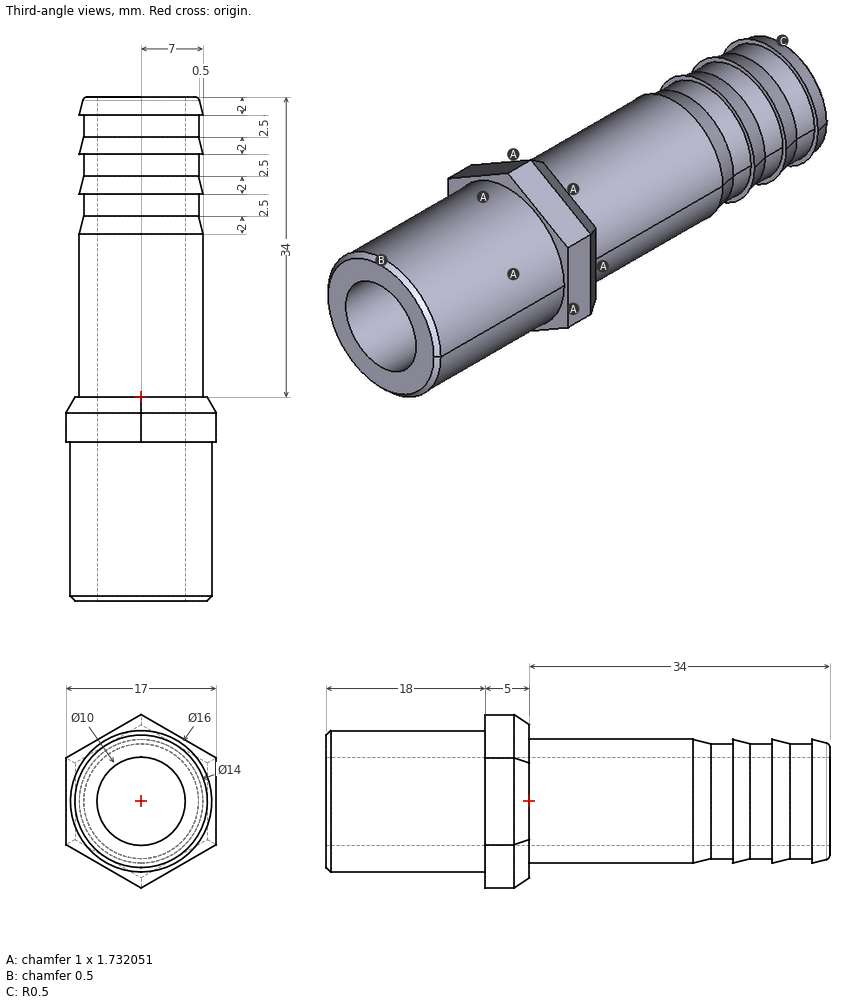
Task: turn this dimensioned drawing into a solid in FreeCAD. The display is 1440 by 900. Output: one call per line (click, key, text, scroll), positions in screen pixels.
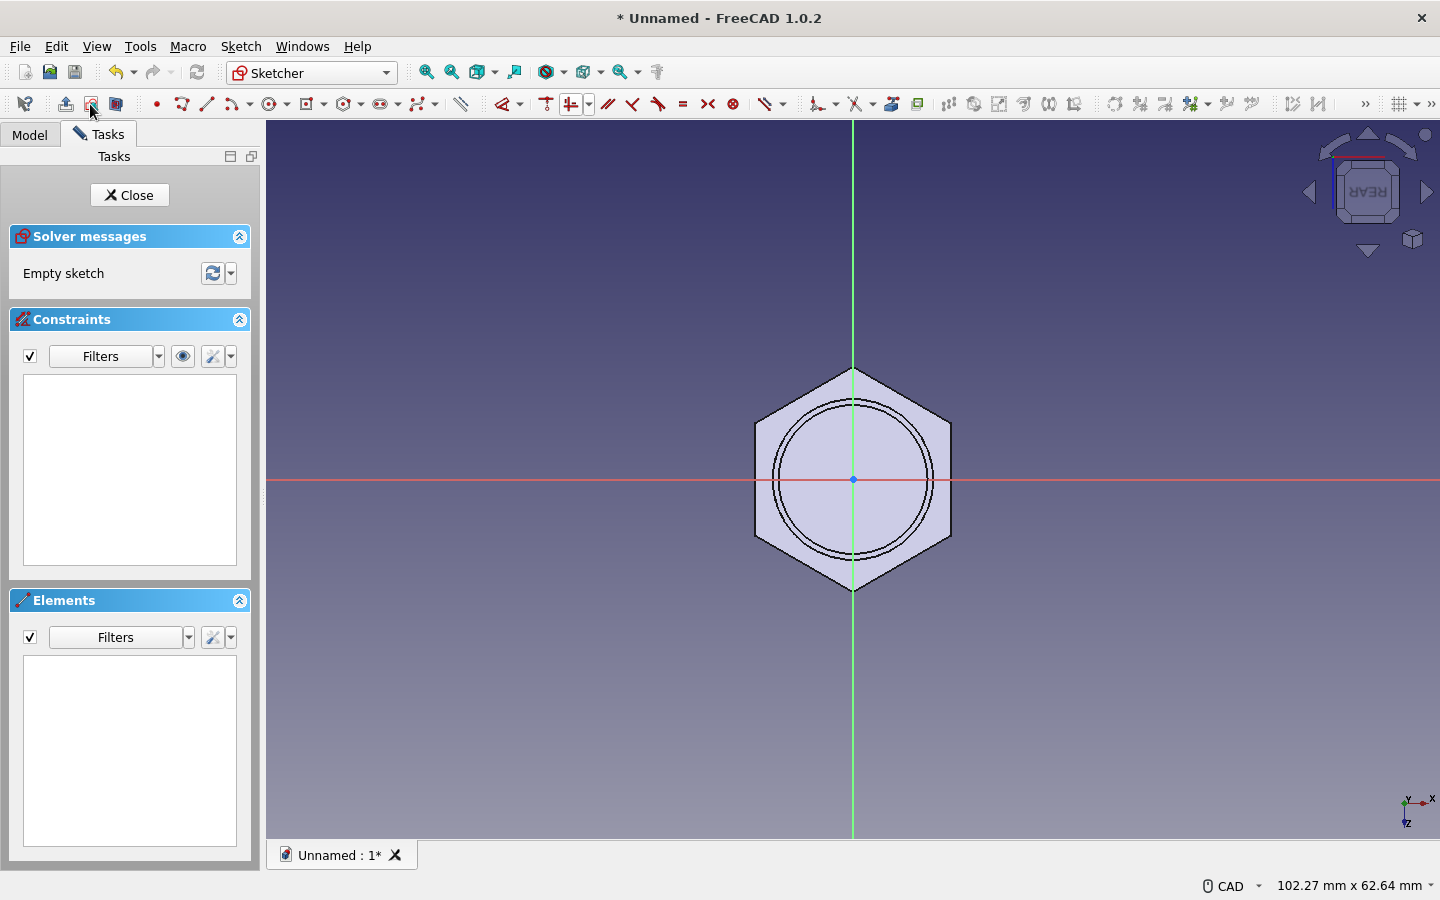
scroll(875, 479, up, 7)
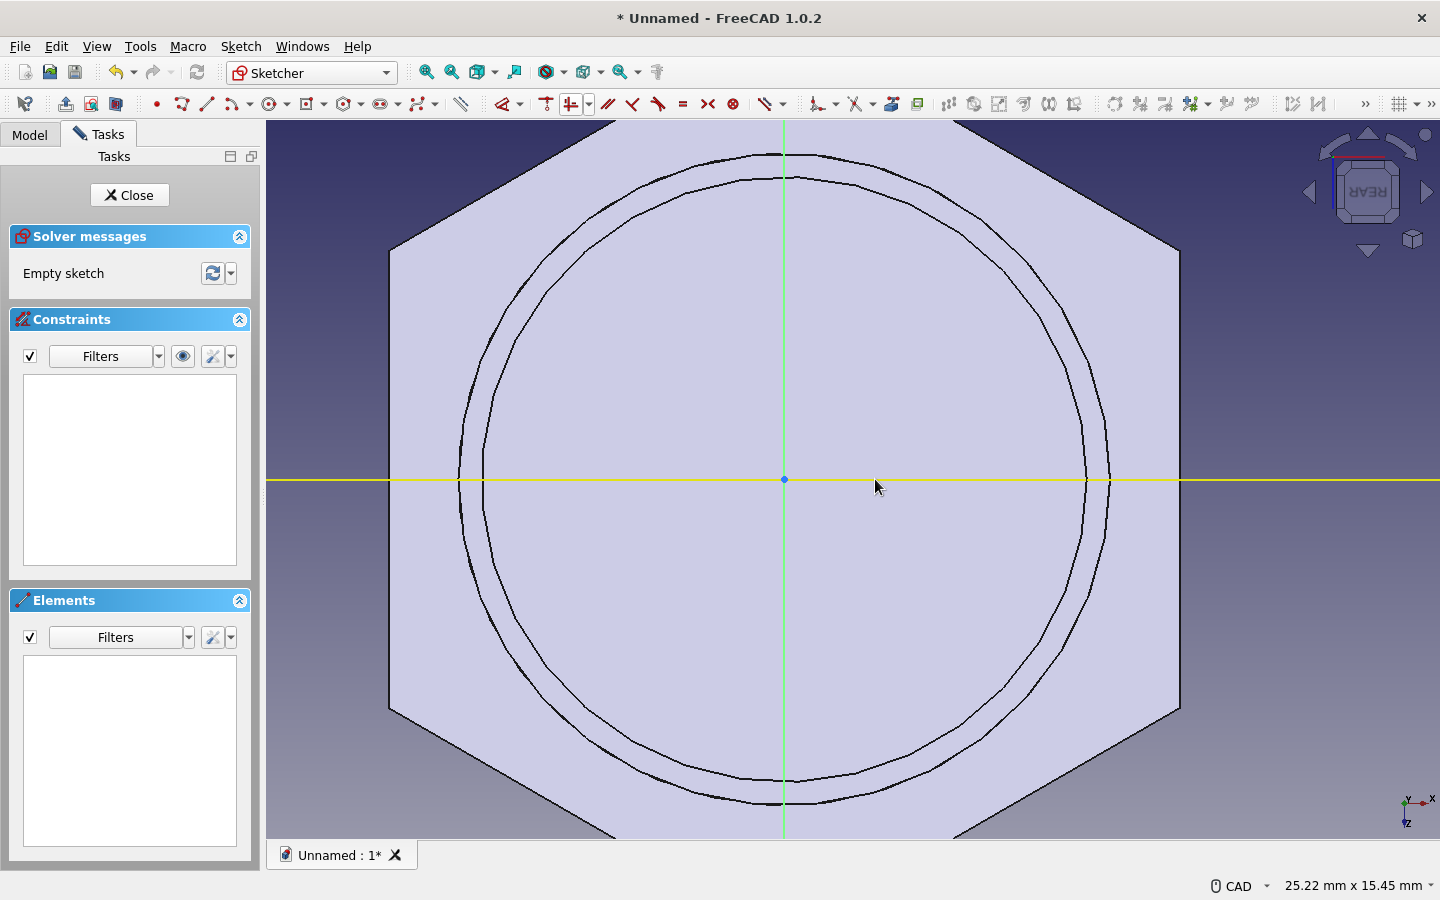
click(268, 104)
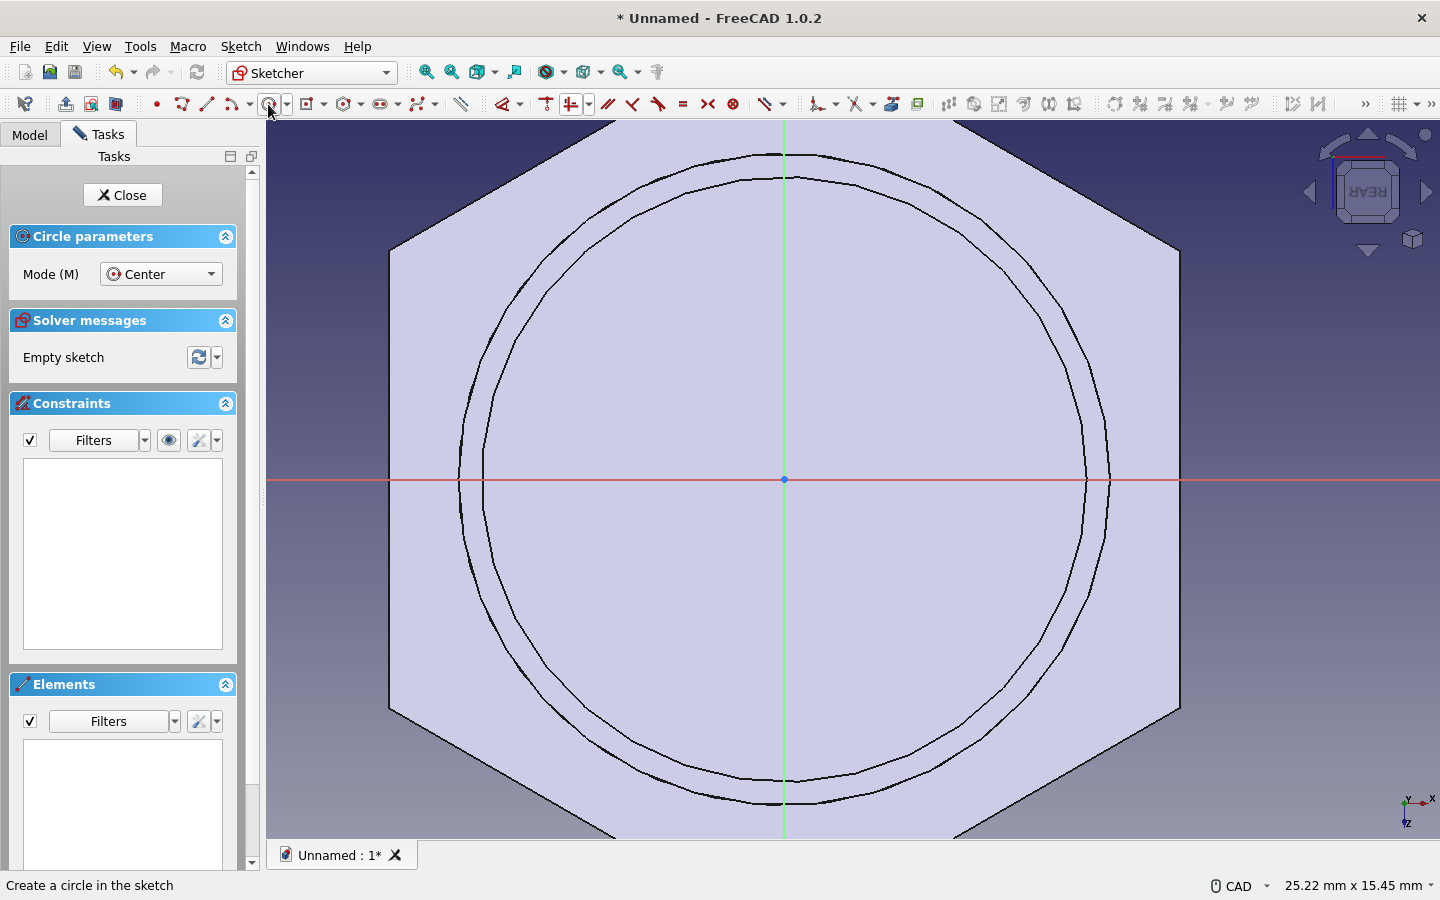
click(784, 479)
click(949, 315)
key(Escape)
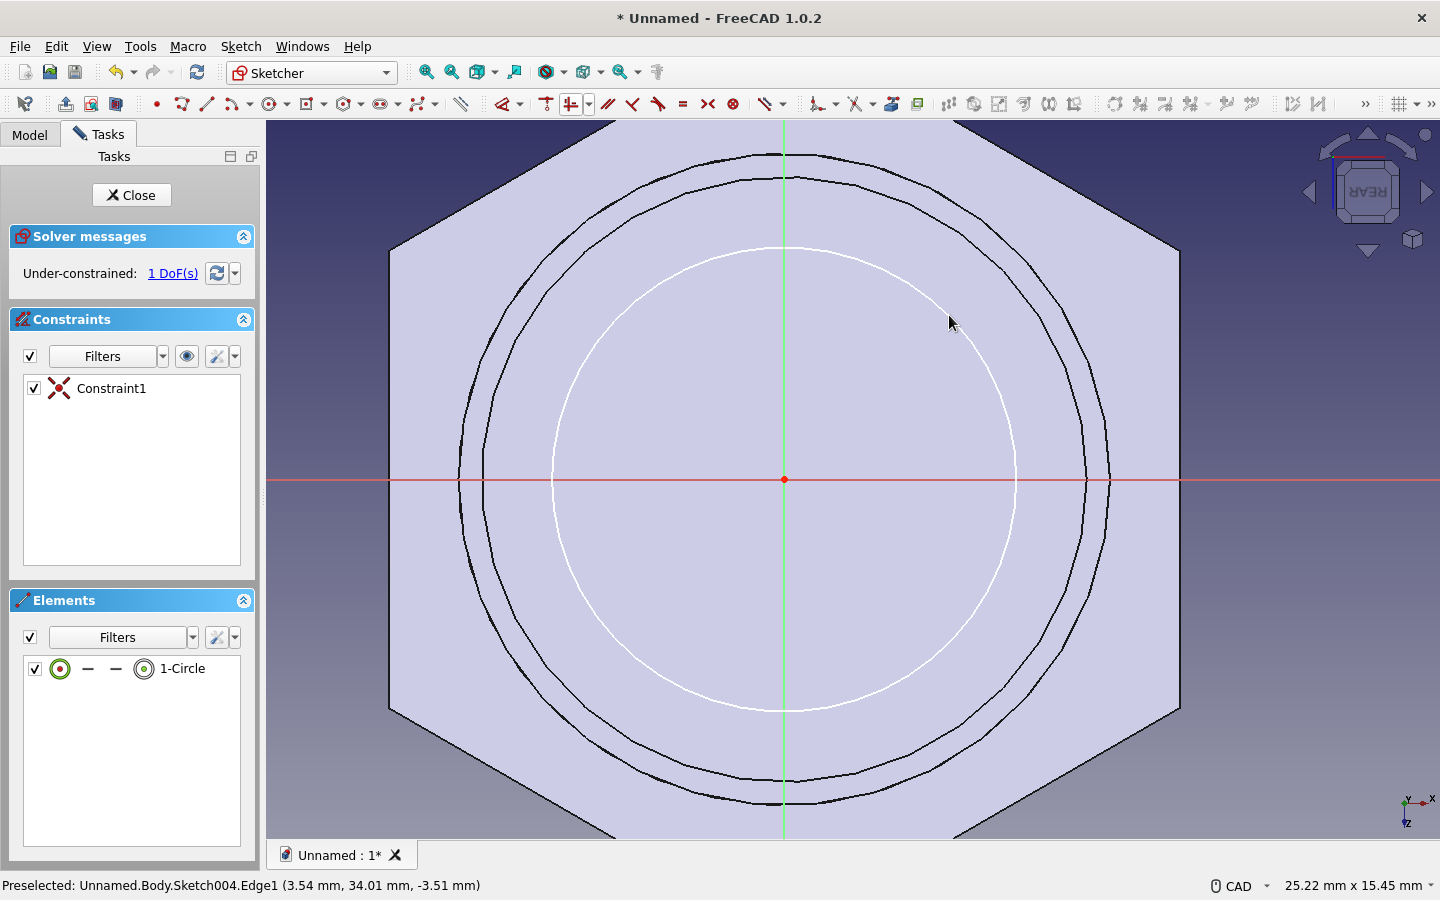
key(d)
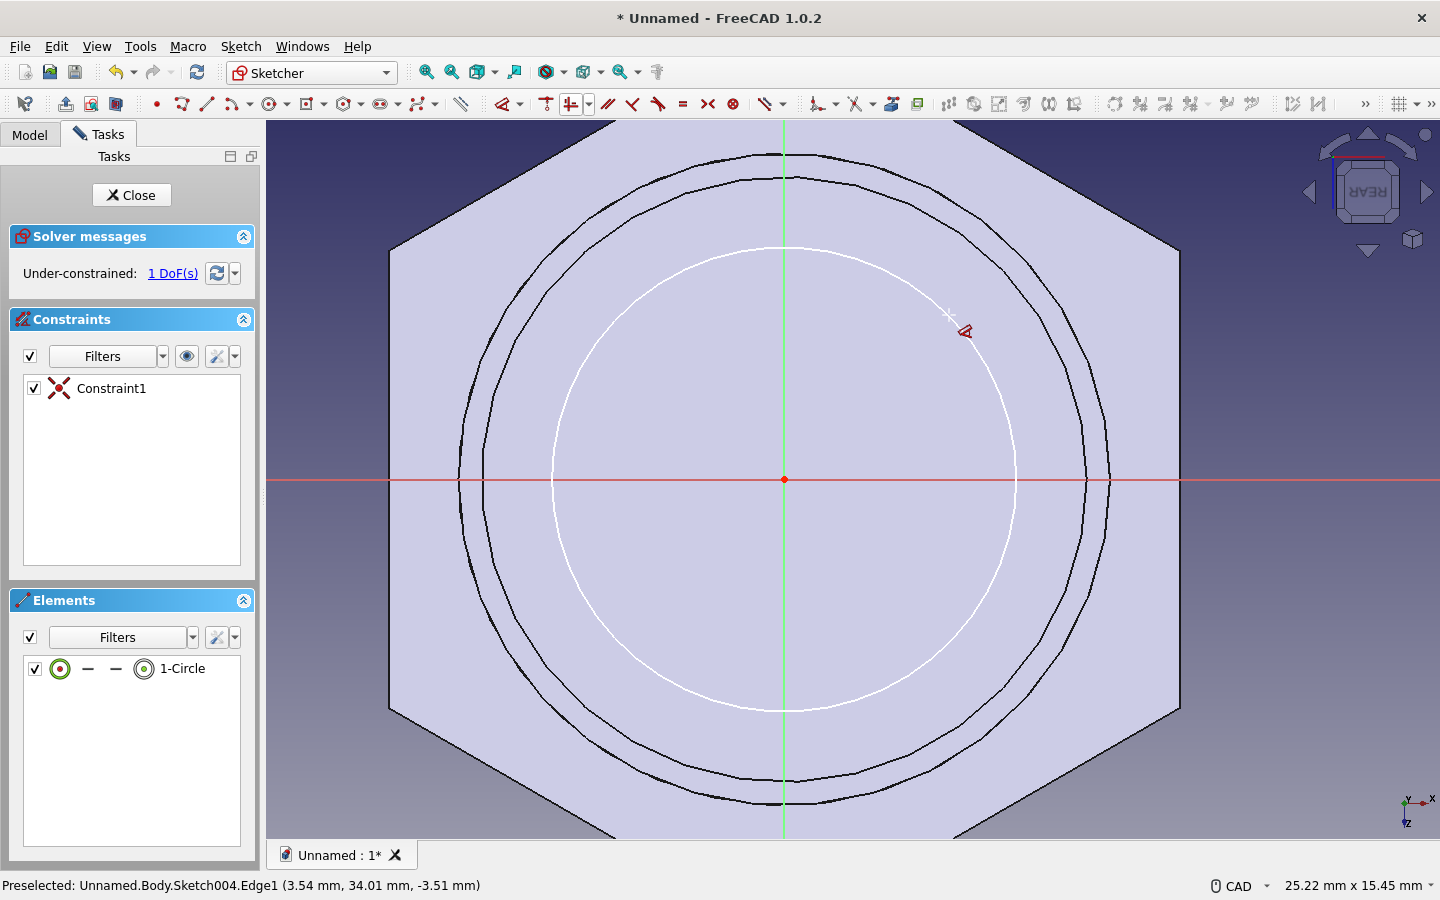
click(948, 315)
click(971, 292)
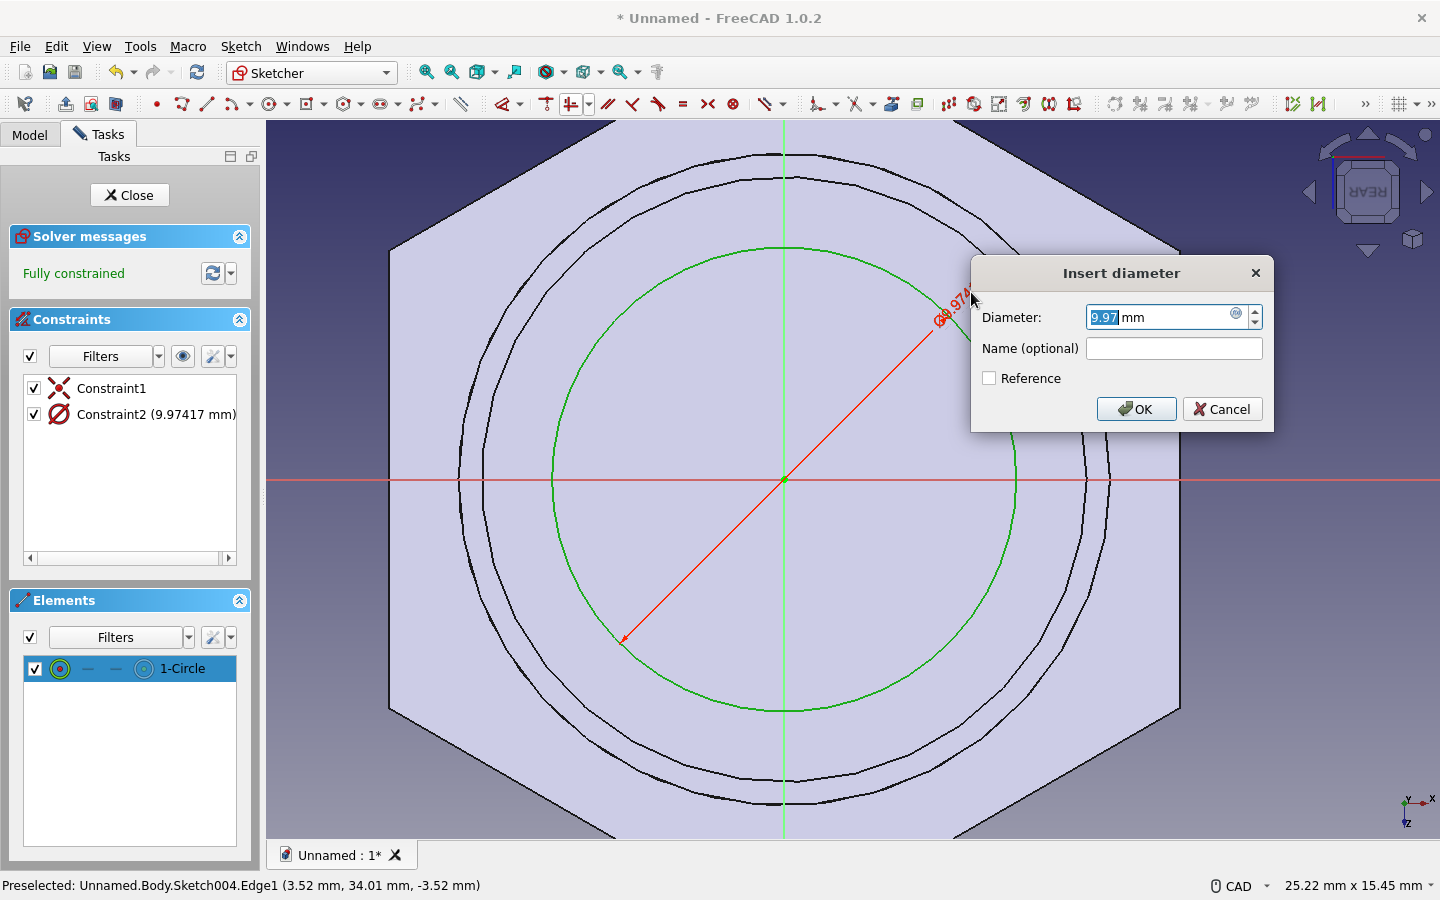
text(10)
key(Return)
key(Escape)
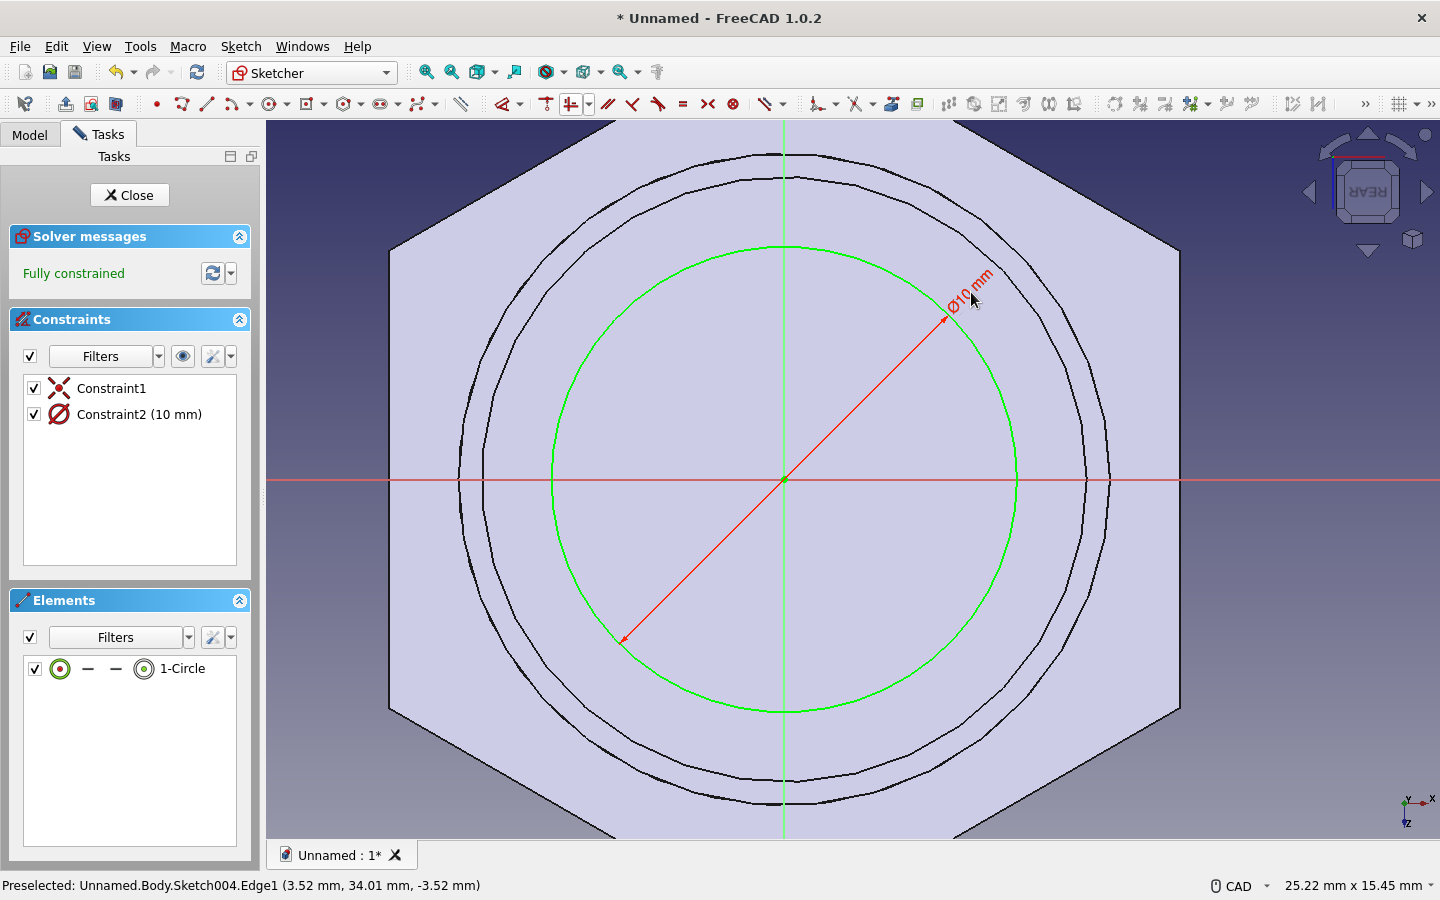
click(130, 195)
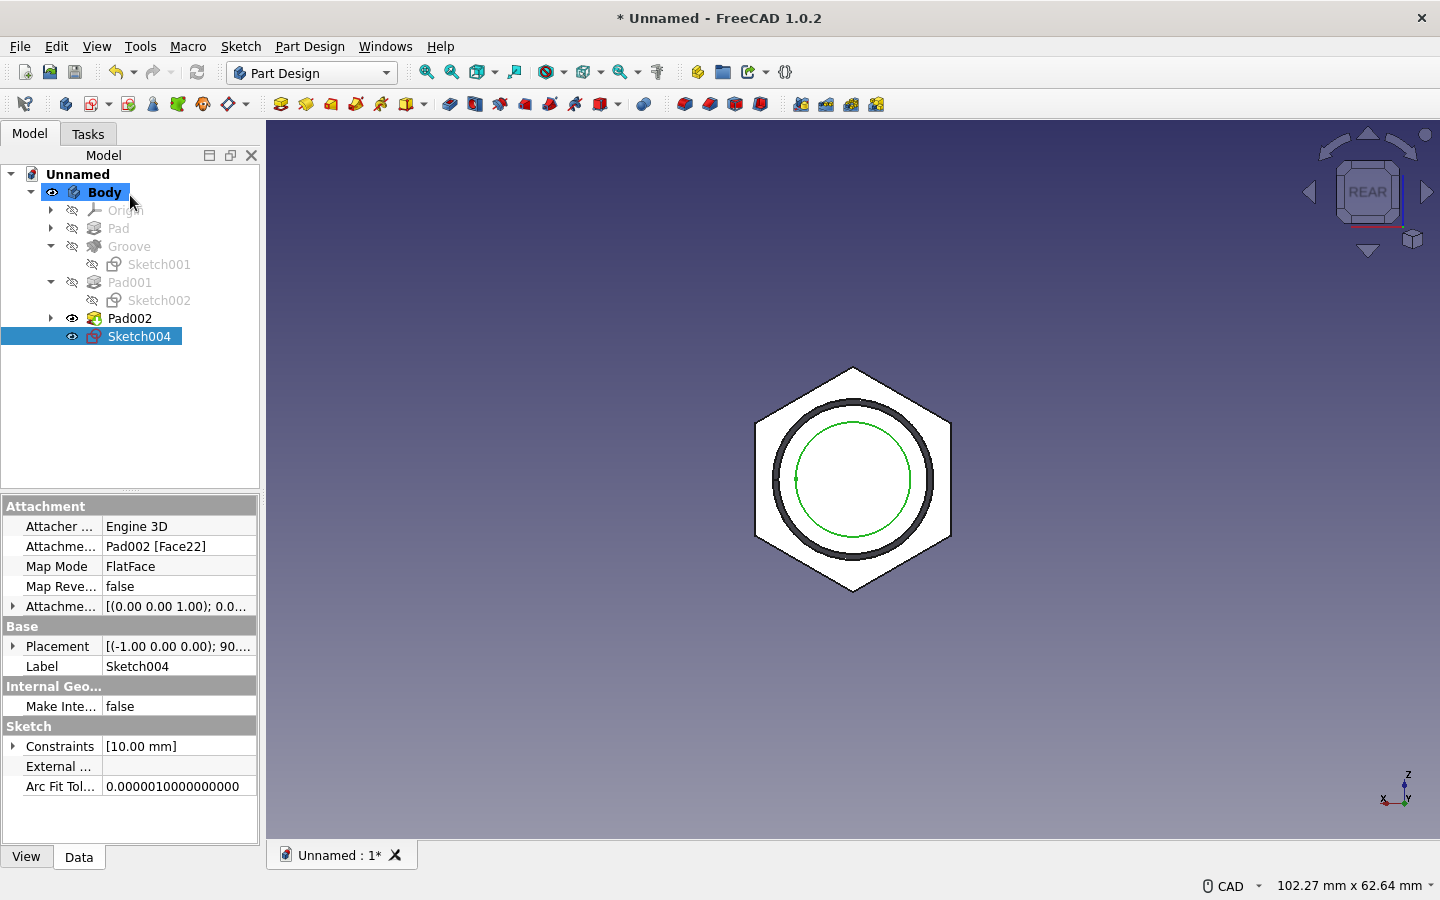
click(450, 104)